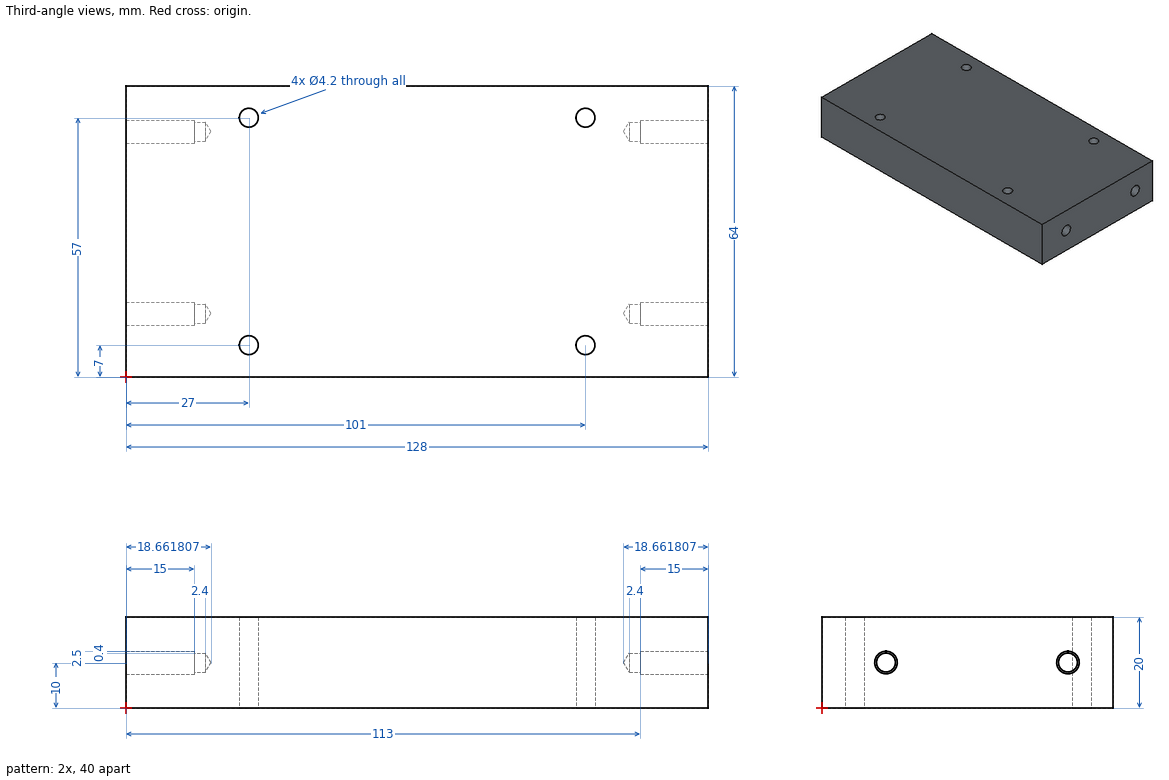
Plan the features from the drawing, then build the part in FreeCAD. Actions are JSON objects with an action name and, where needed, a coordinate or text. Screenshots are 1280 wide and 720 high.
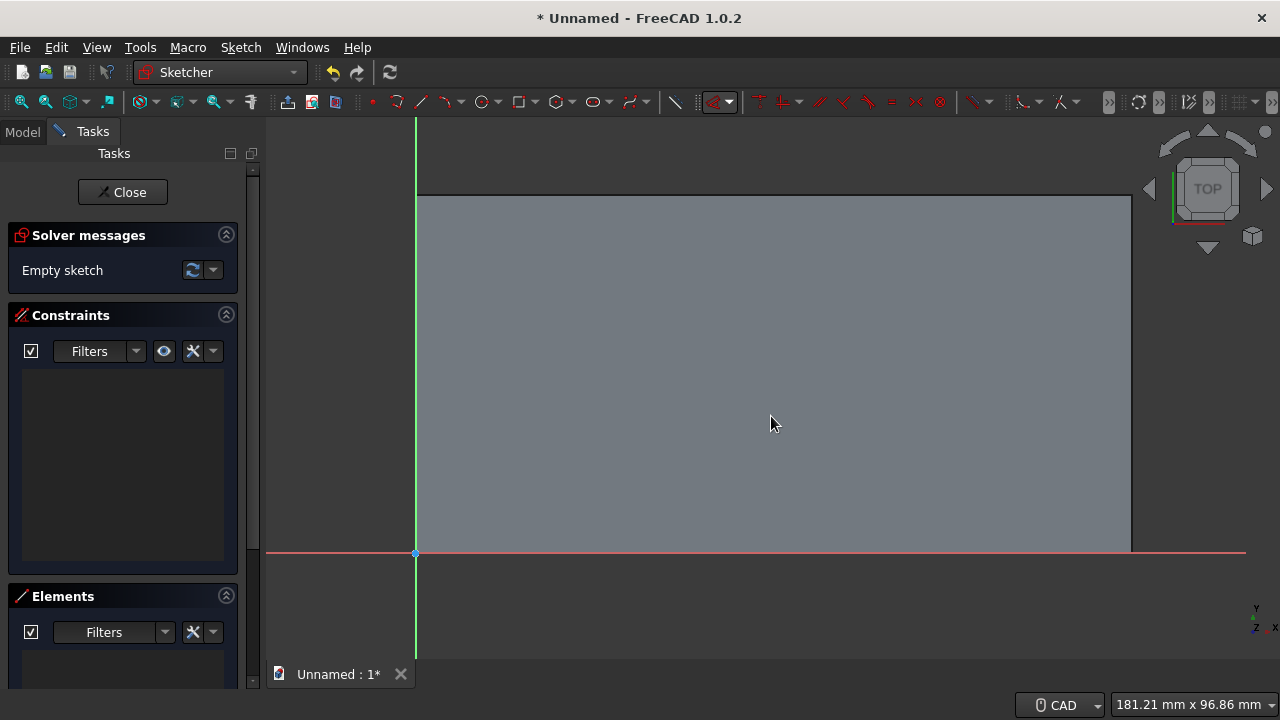
{"action": "left_click", "coordinate": [482, 102]}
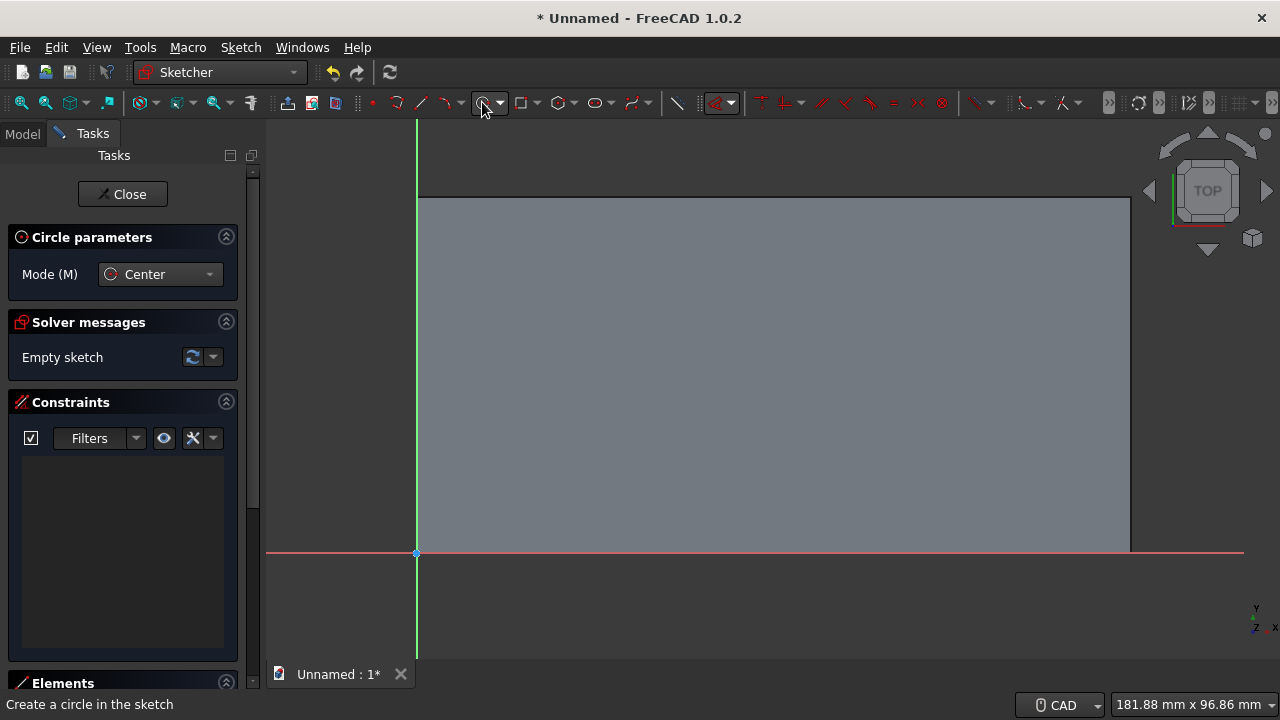
{"action": "scroll", "coordinate": [567, 236], "scroll_direction": "up", "scroll_amount": 4}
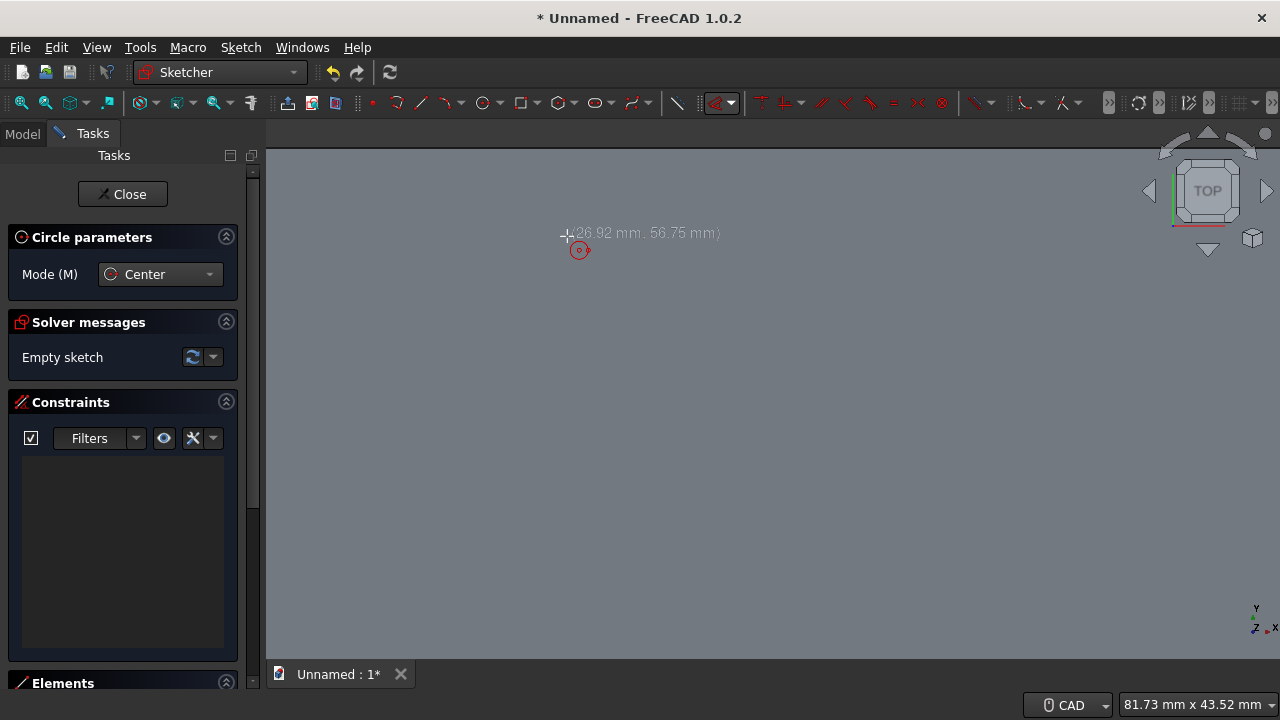
{"action": "left_click", "coordinate": [568, 235]}
{"action": "left_click", "coordinate": [586, 216]}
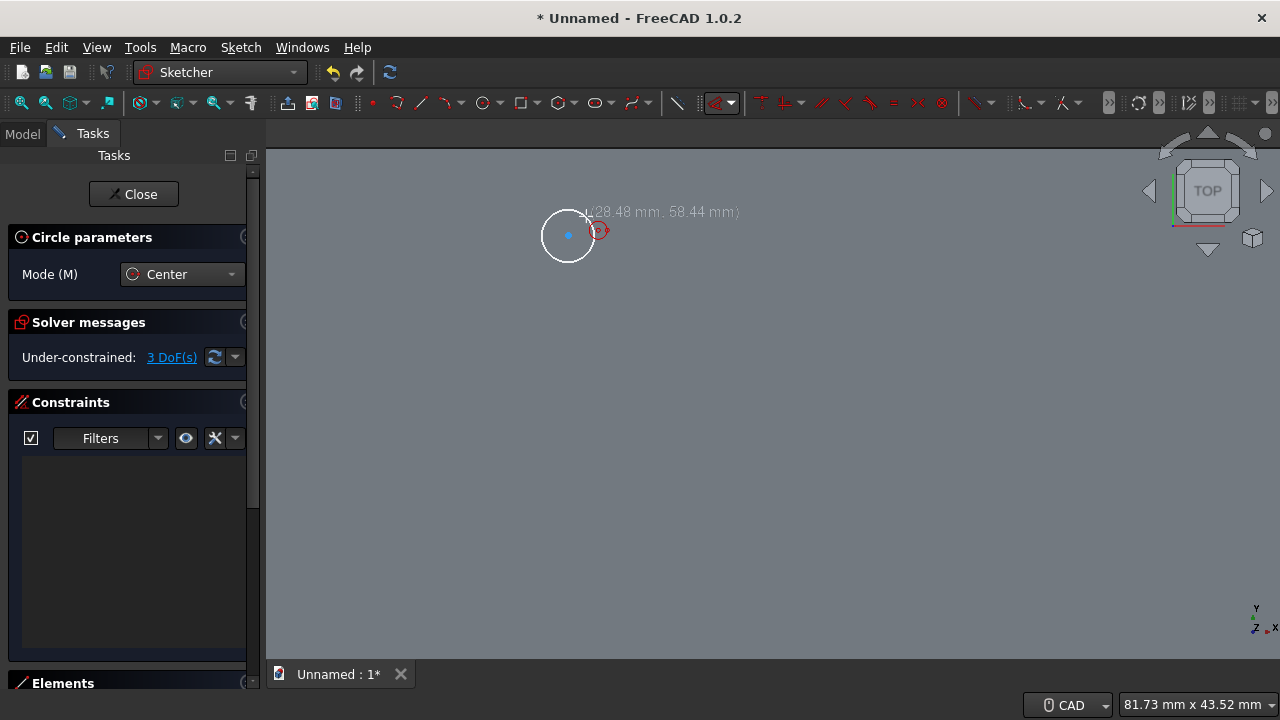
{"action": "scroll", "coordinate": [568, 237], "scroll_direction": "down", "scroll_amount": 4}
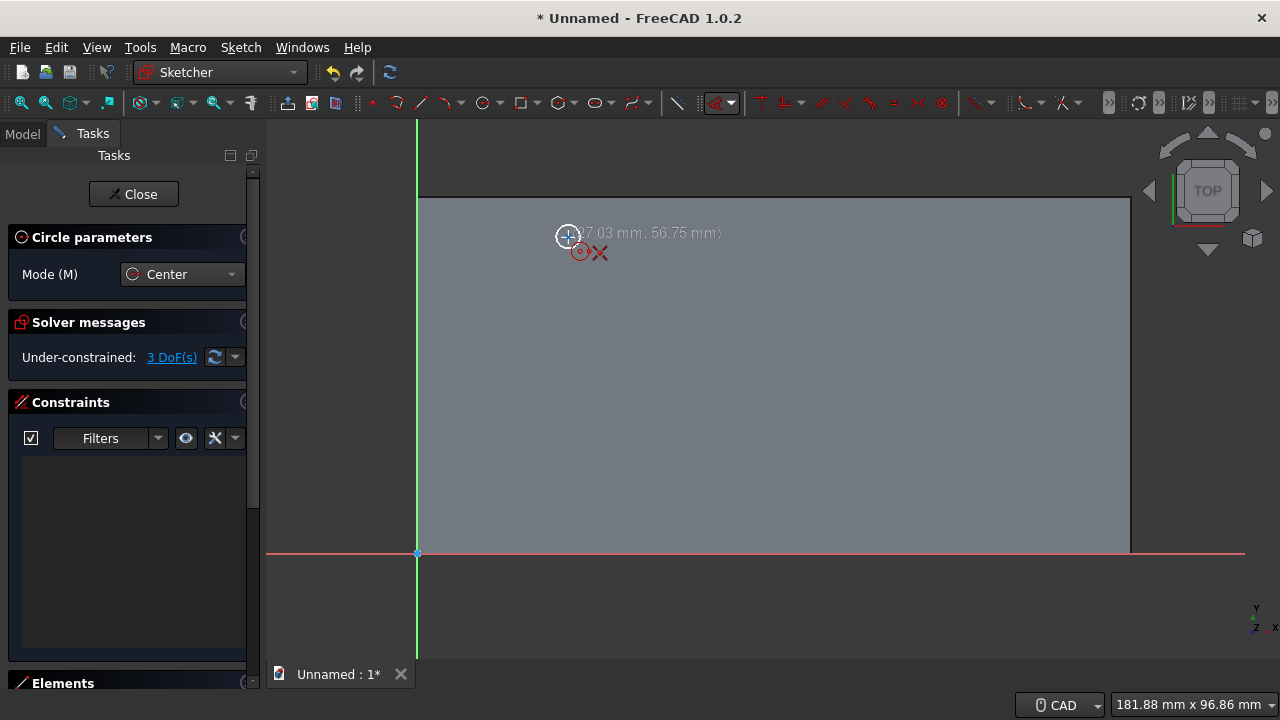
{"action": "scroll", "coordinate": [568, 515], "scroll_direction": "up", "scroll_amount": 4}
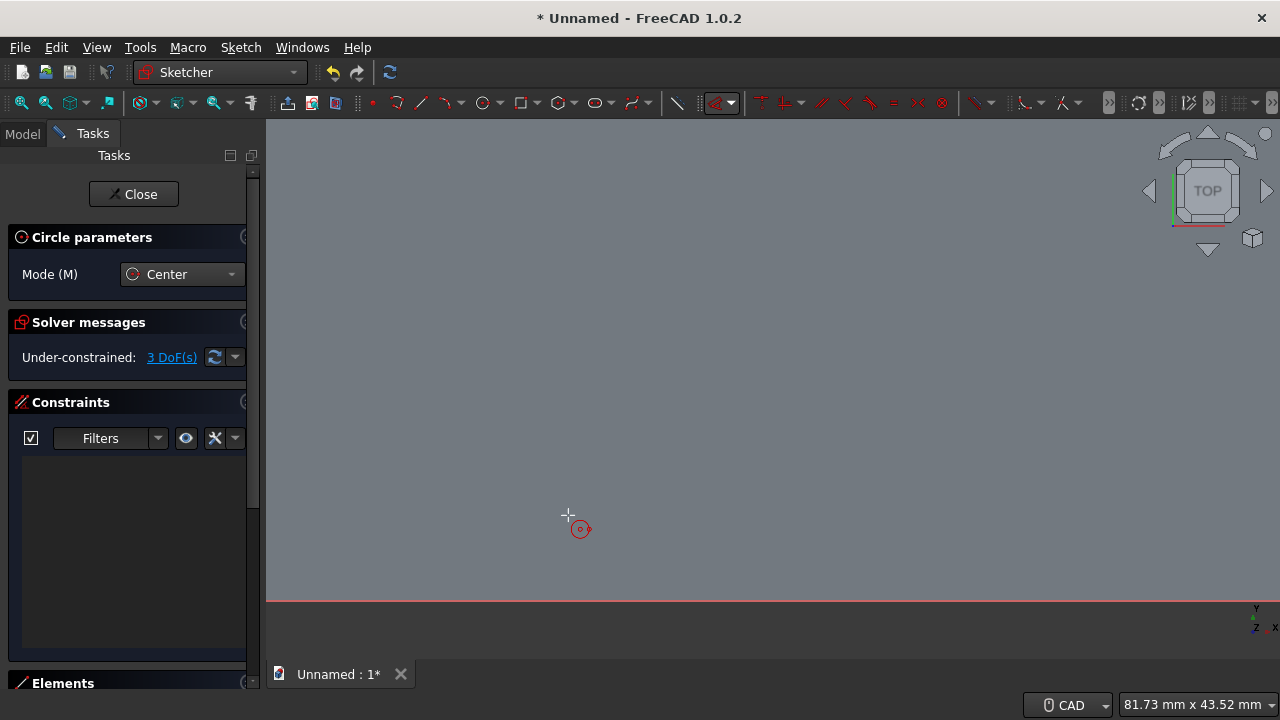
{"action": "left_click", "coordinate": [568, 514]}
{"action": "left_click", "coordinate": [586, 496]}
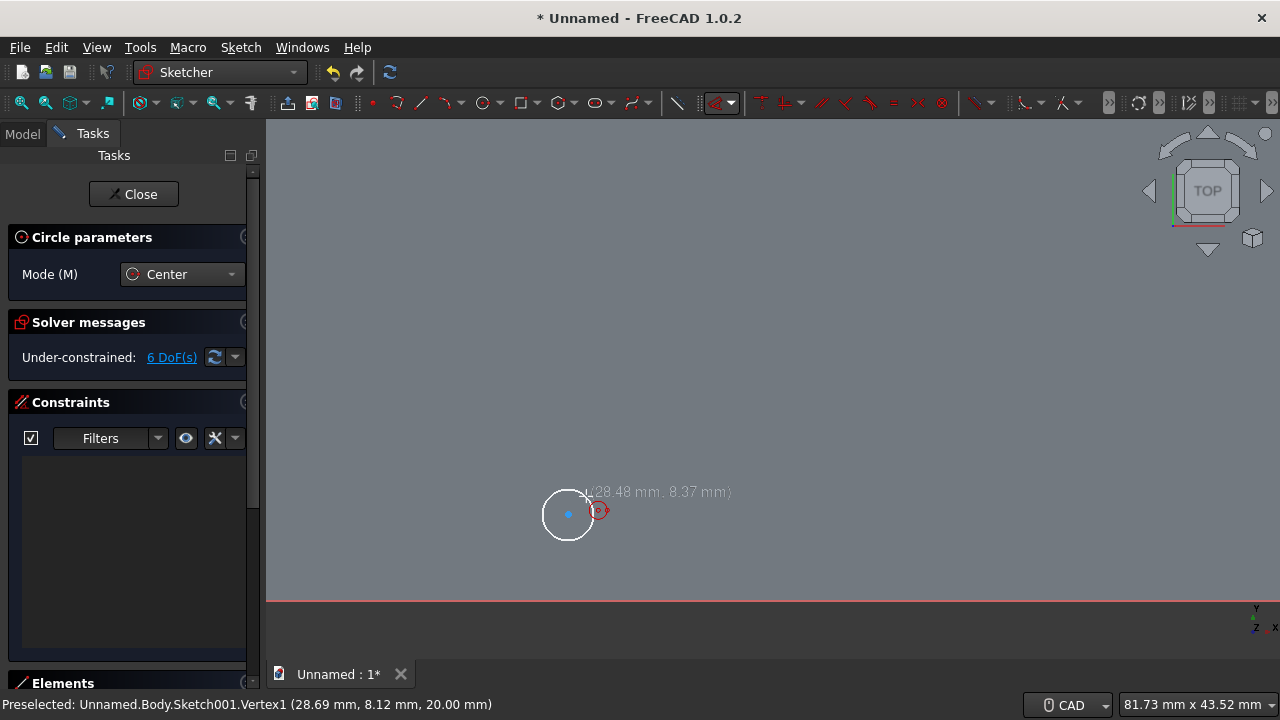
{"action": "scroll", "coordinate": [568, 515], "scroll_direction": "down", "scroll_amount": 4}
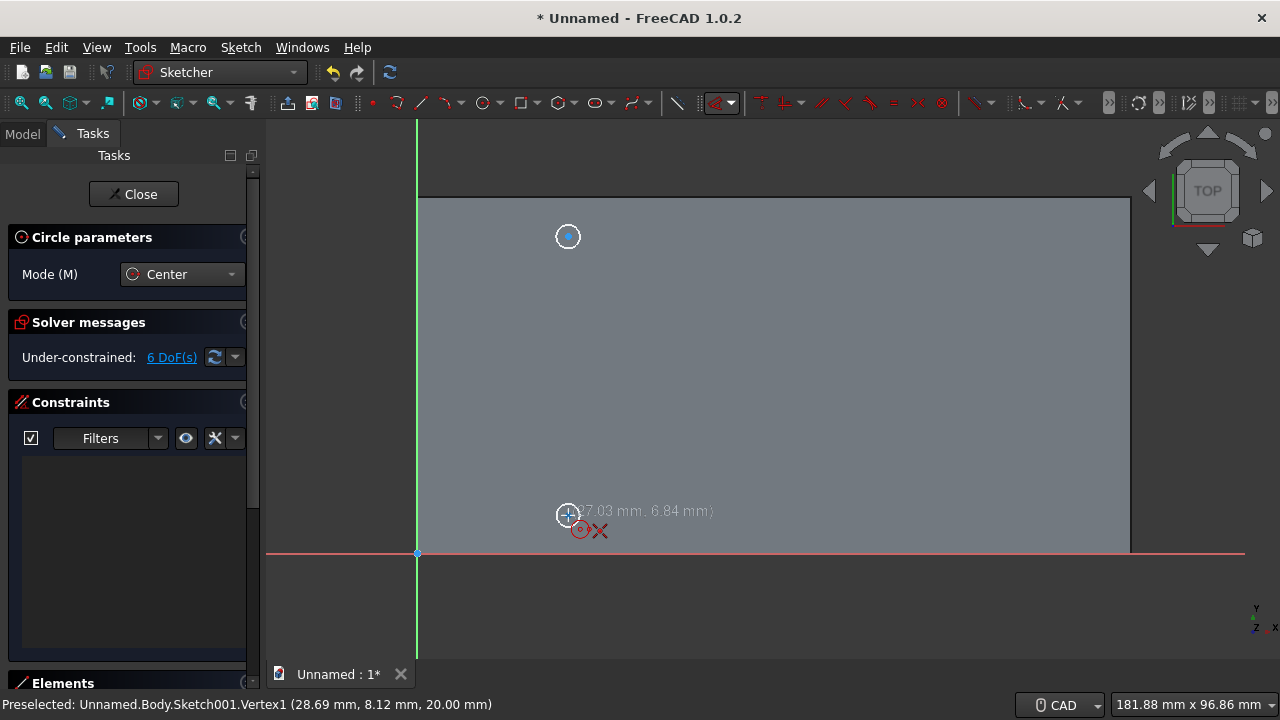
{"action": "scroll", "coordinate": [981, 515], "scroll_direction": "up", "scroll_amount": 4}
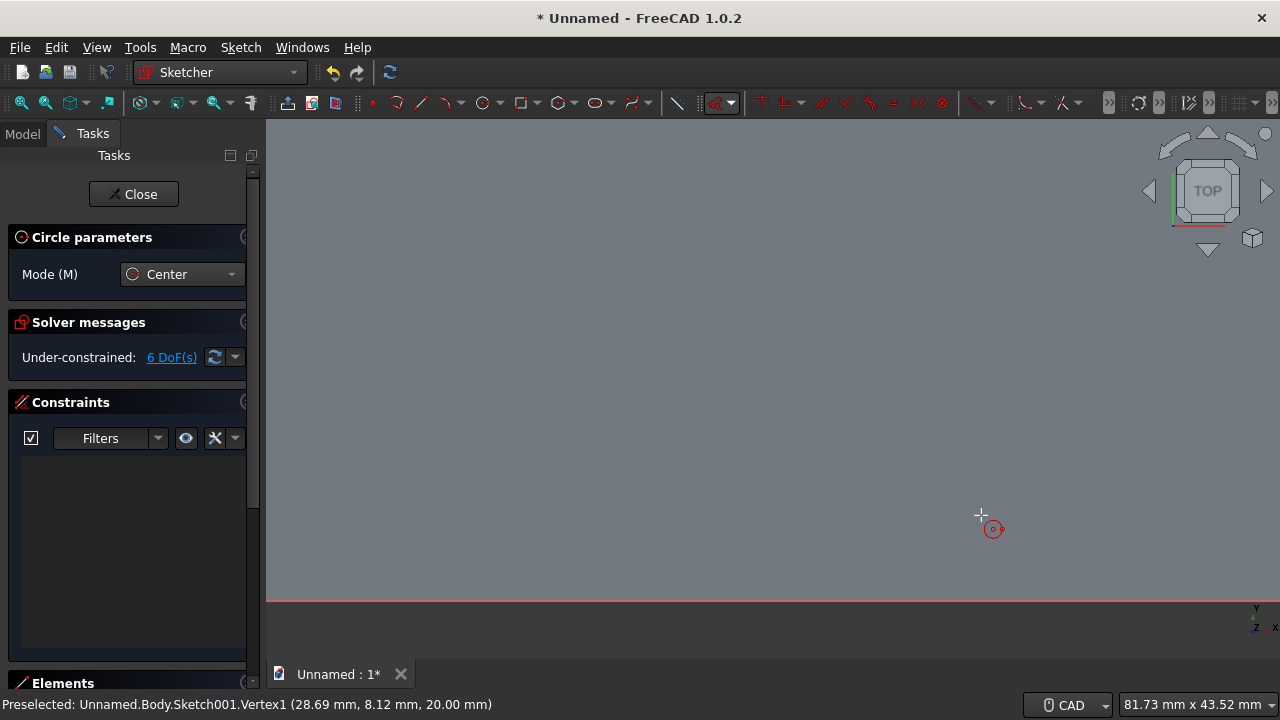
{"action": "left_click", "coordinate": [979, 514]}
{"action": "left_click", "coordinate": [998, 496]}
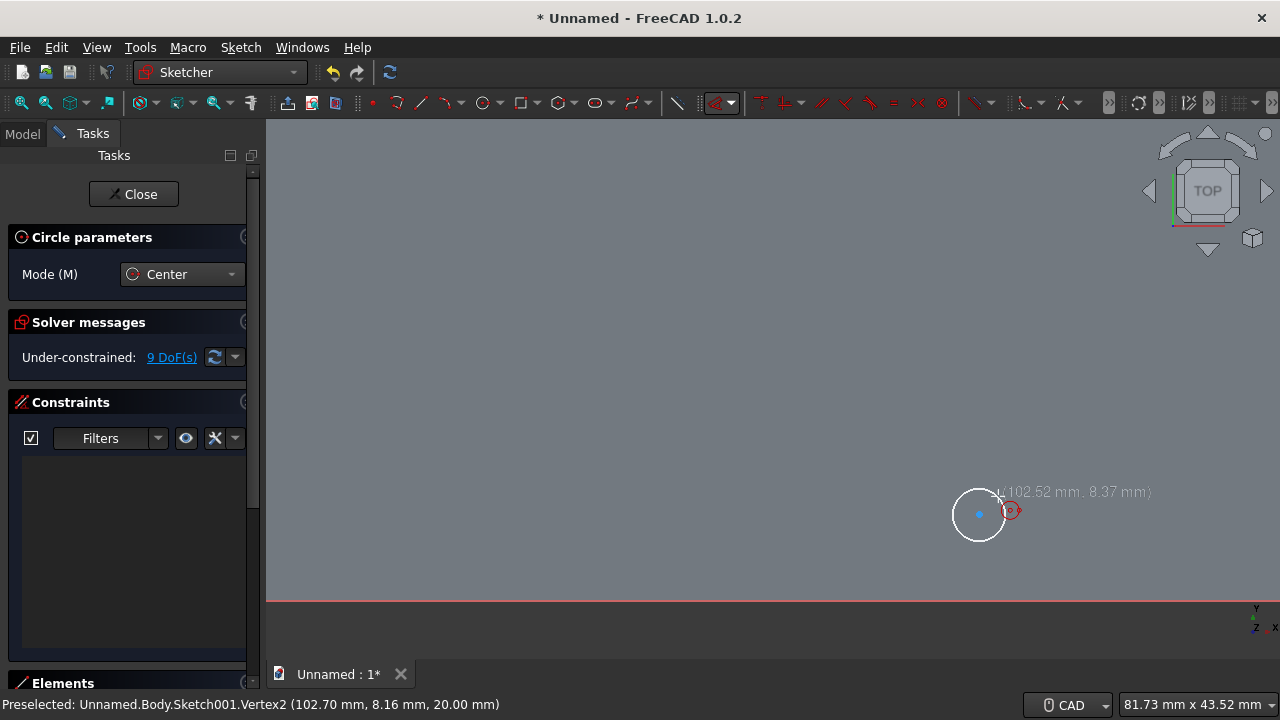
{"action": "scroll", "coordinate": [981, 515], "scroll_direction": "down", "scroll_amount": 4}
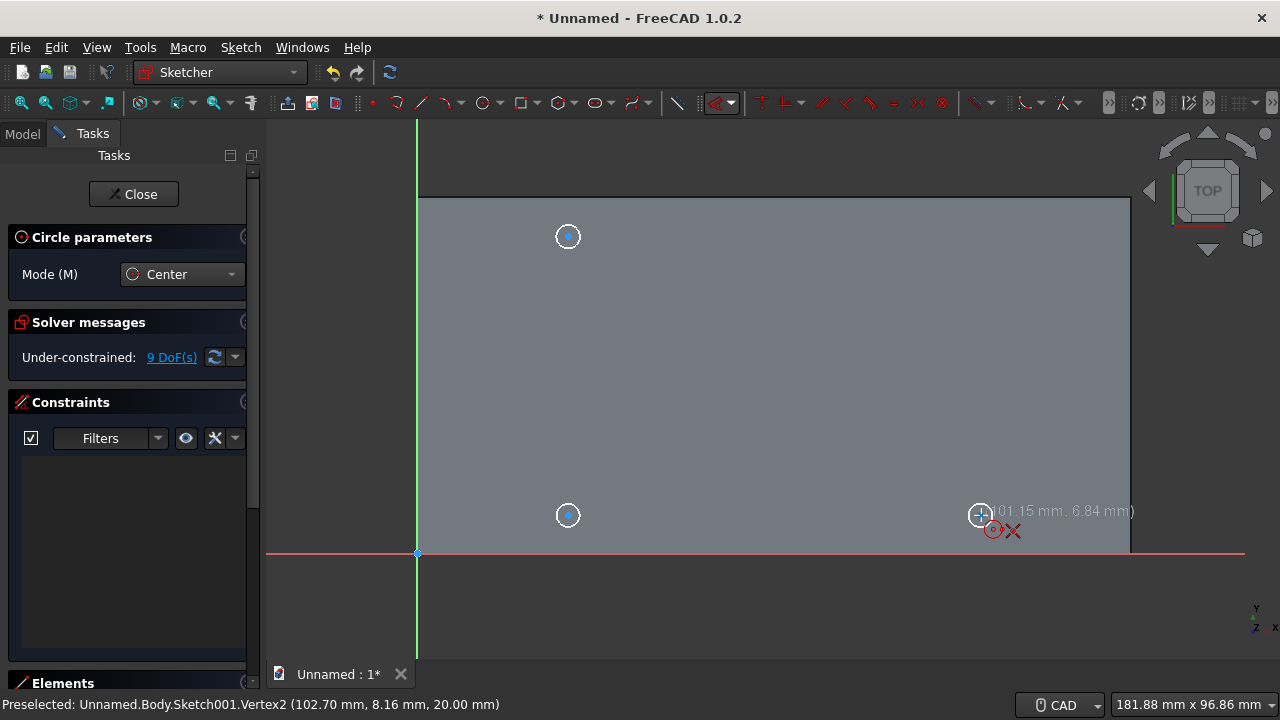
{"action": "scroll", "coordinate": [981, 236], "scroll_direction": "up", "scroll_amount": 4}